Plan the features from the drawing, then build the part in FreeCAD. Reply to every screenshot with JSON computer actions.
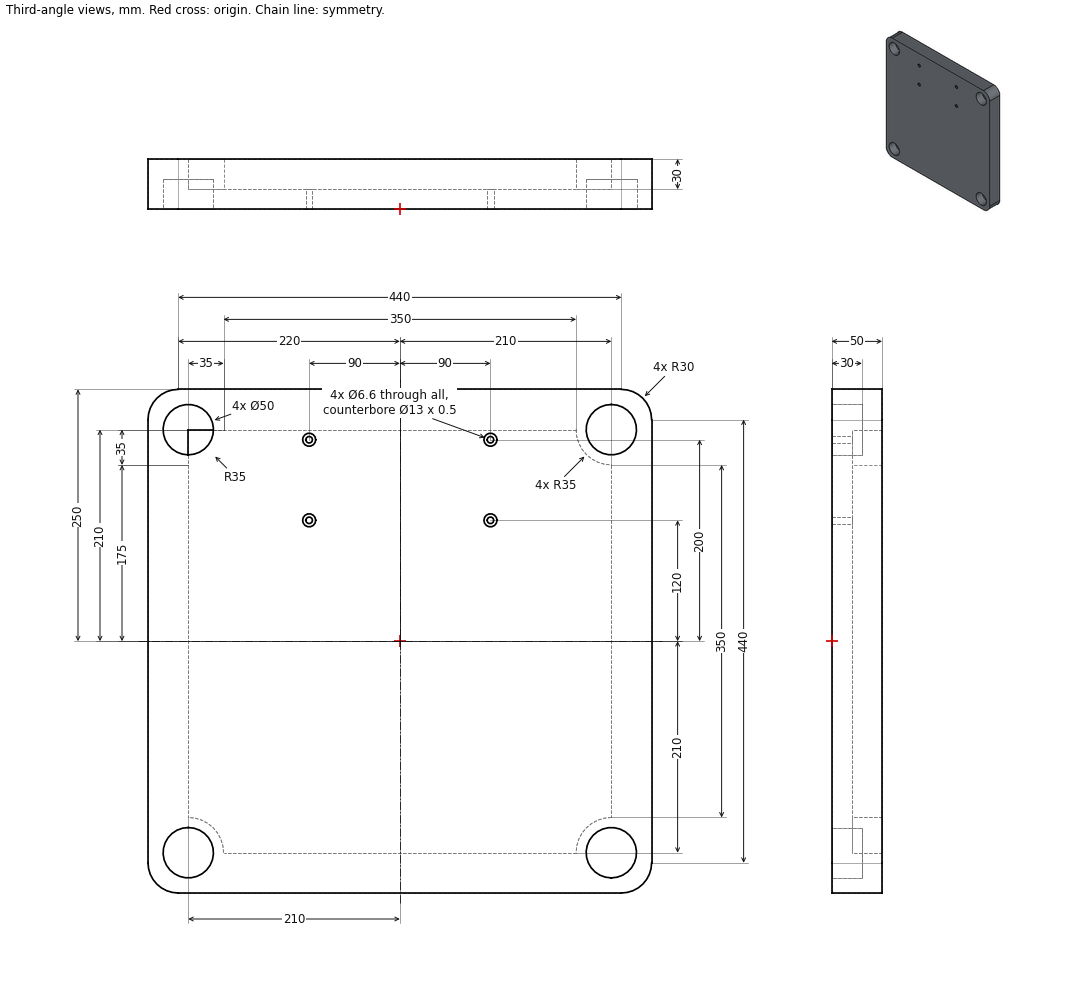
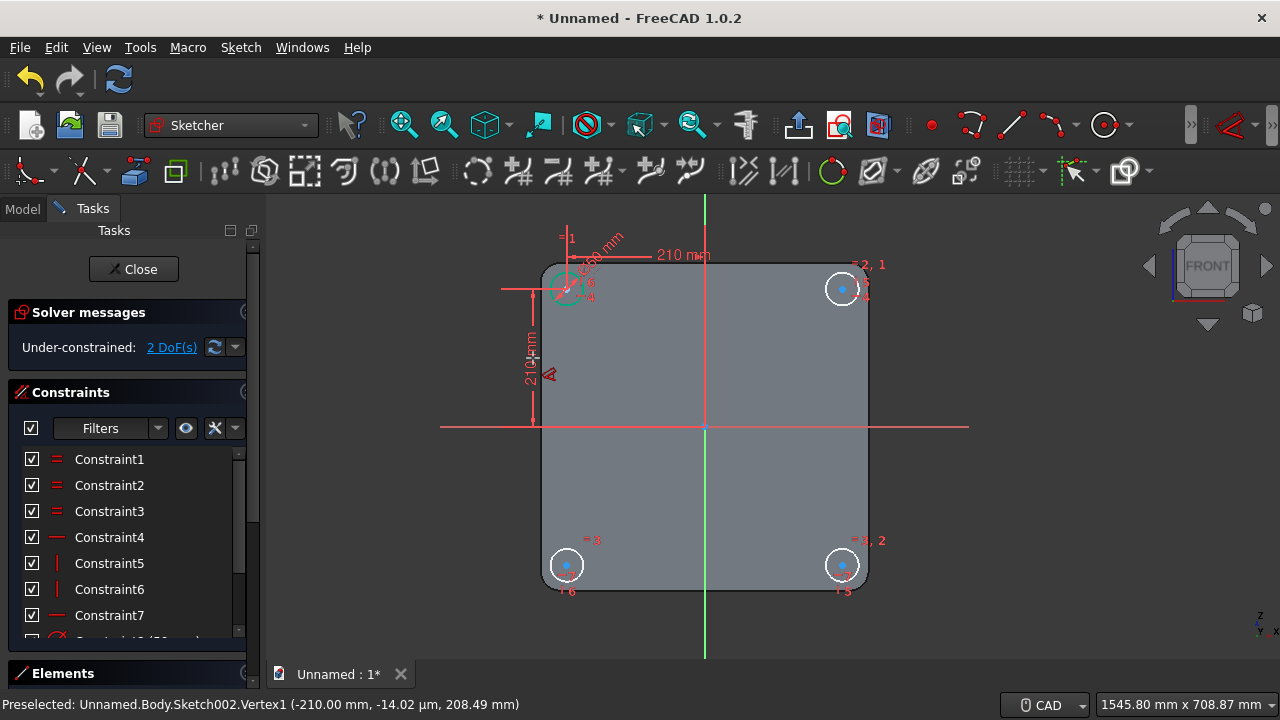
{"action": "left_click", "coordinate": [842, 289]}
{"action": "left_click", "coordinate": [773, 255]}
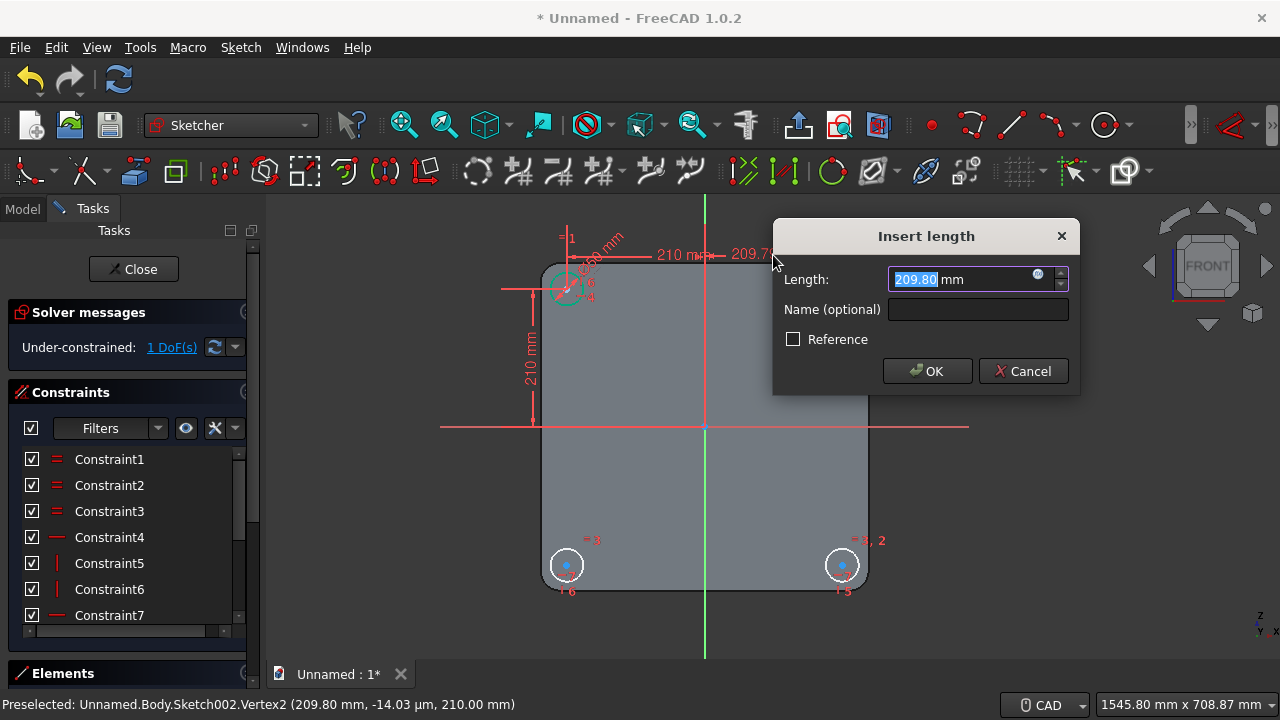
{"action": "type", "text": "210"}
{"action": "key", "text": "Return"}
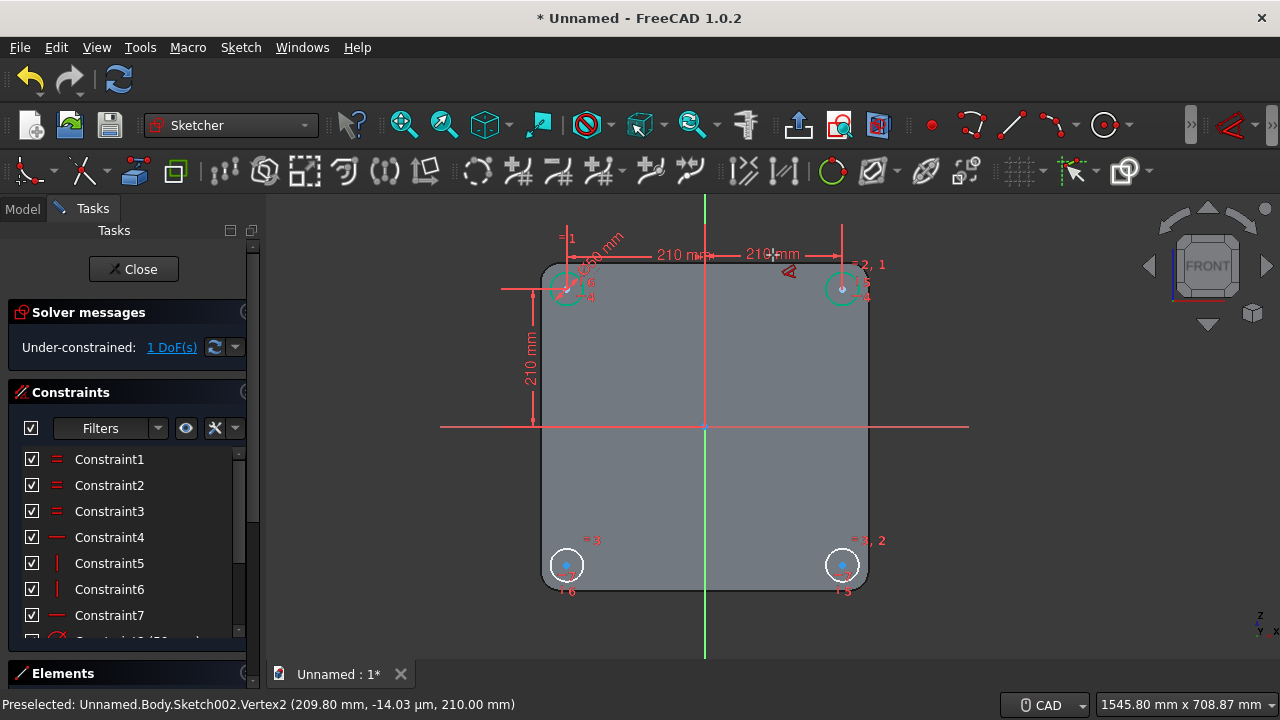
{"action": "left_click", "coordinate": [842, 565]}
{"action": "left_click", "coordinate": [876, 496]}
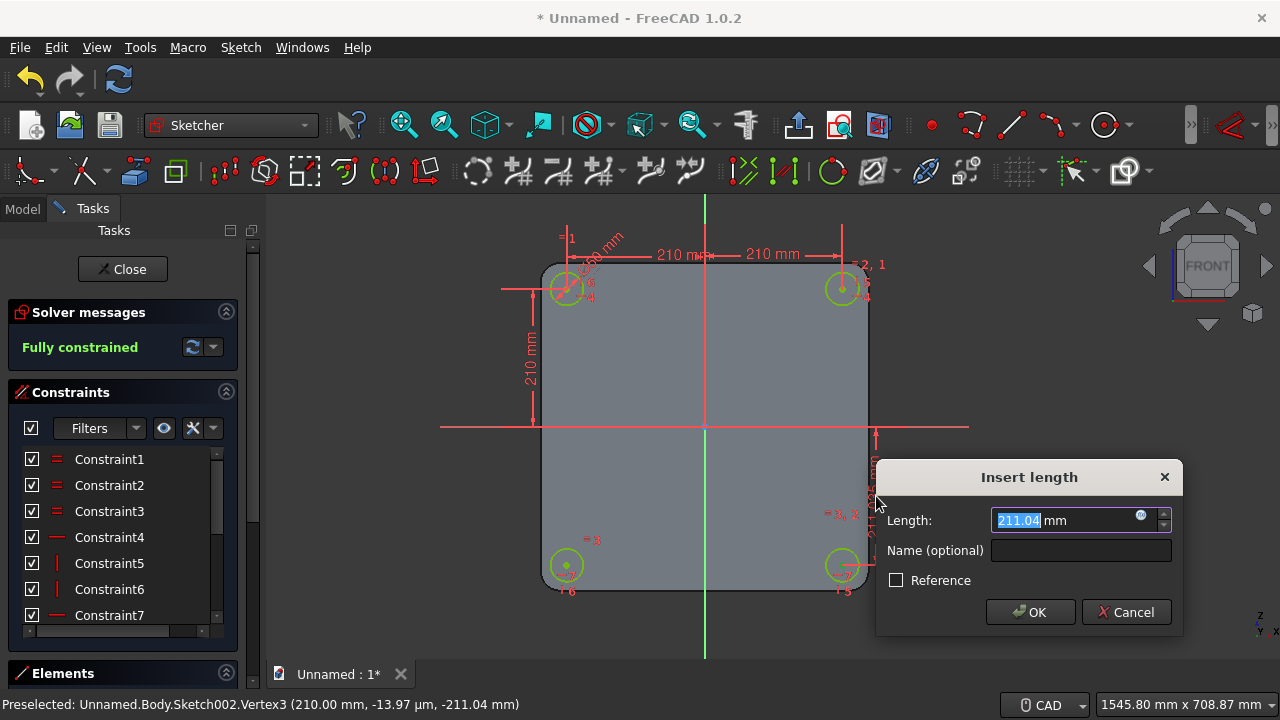
{"action": "type", "text": "210"}
{"action": "key", "text": "Return"}
{"action": "key", "text": "Escape"}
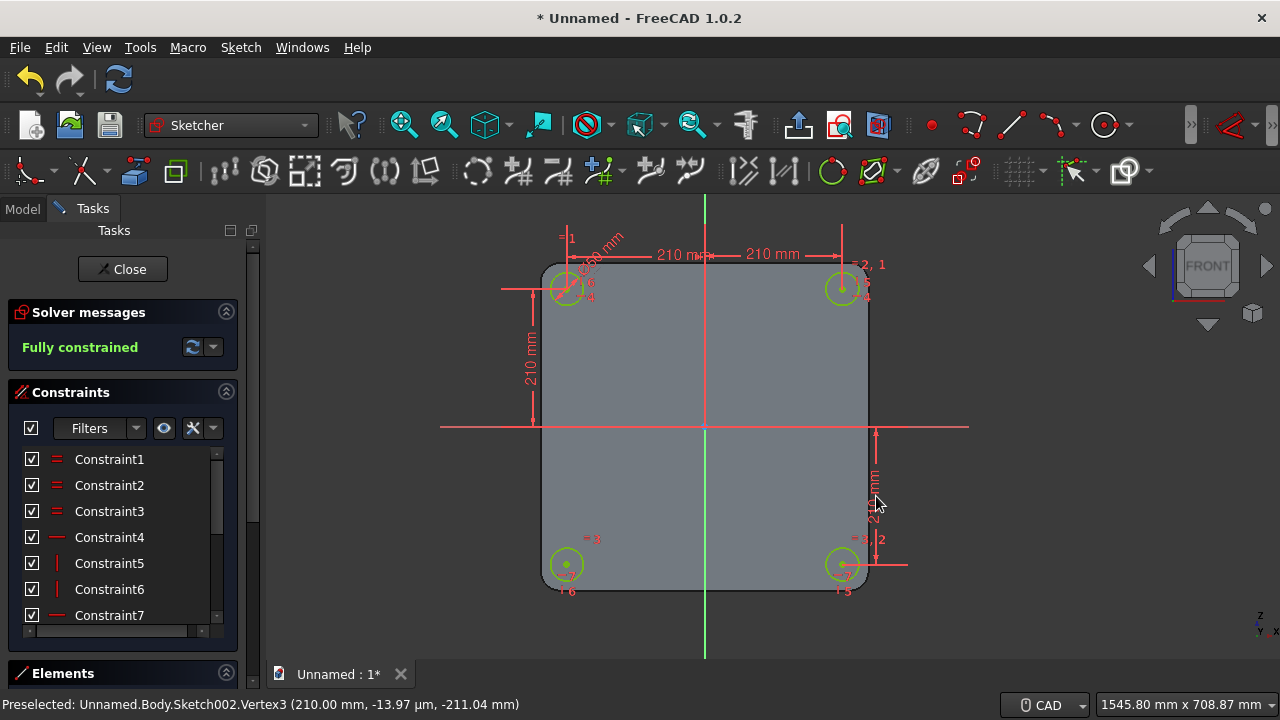
{"action": "left_click", "coordinate": [123, 269]}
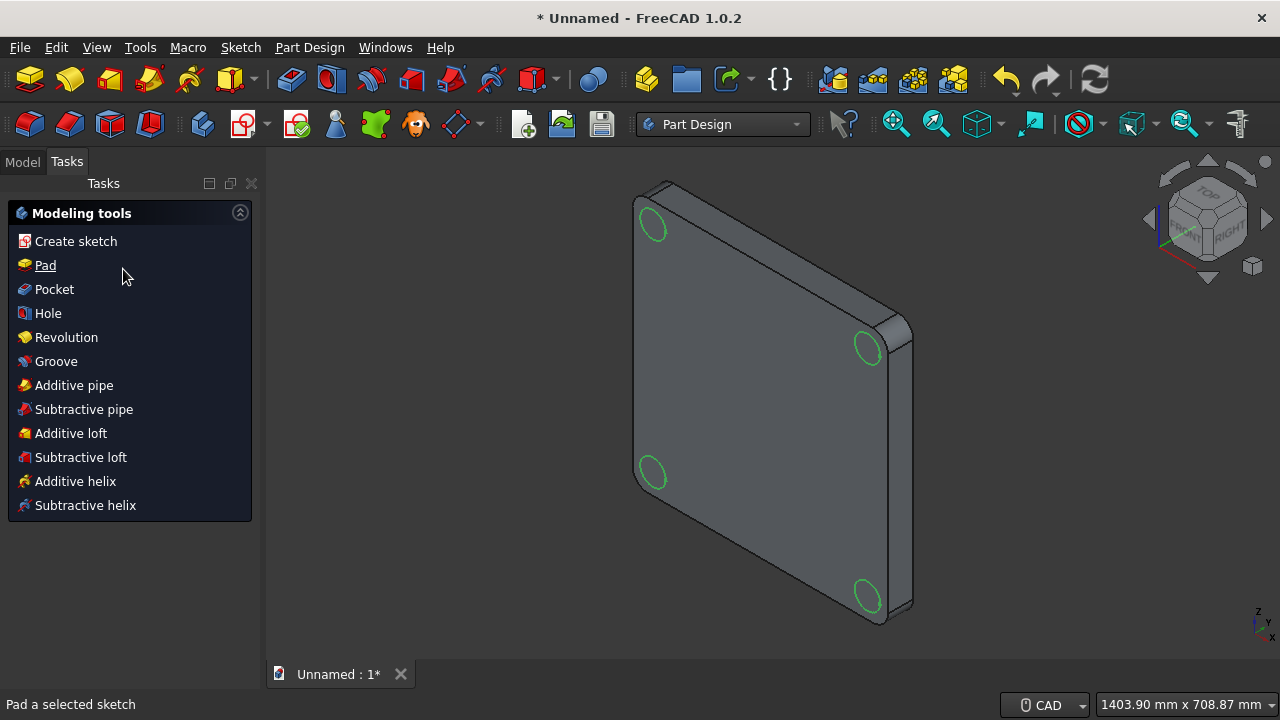
{"action": "left_click", "coordinate": [292, 80]}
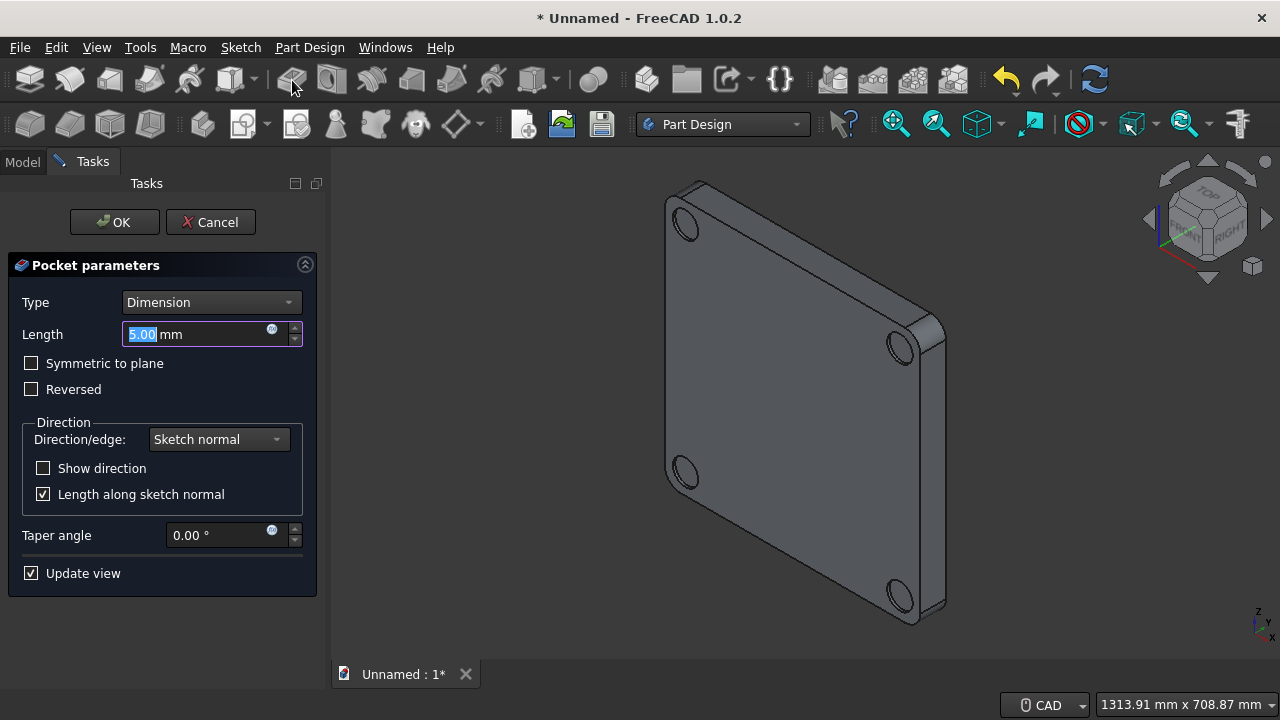
{"action": "type", "text": "30"}
{"action": "key", "text": "Tab"}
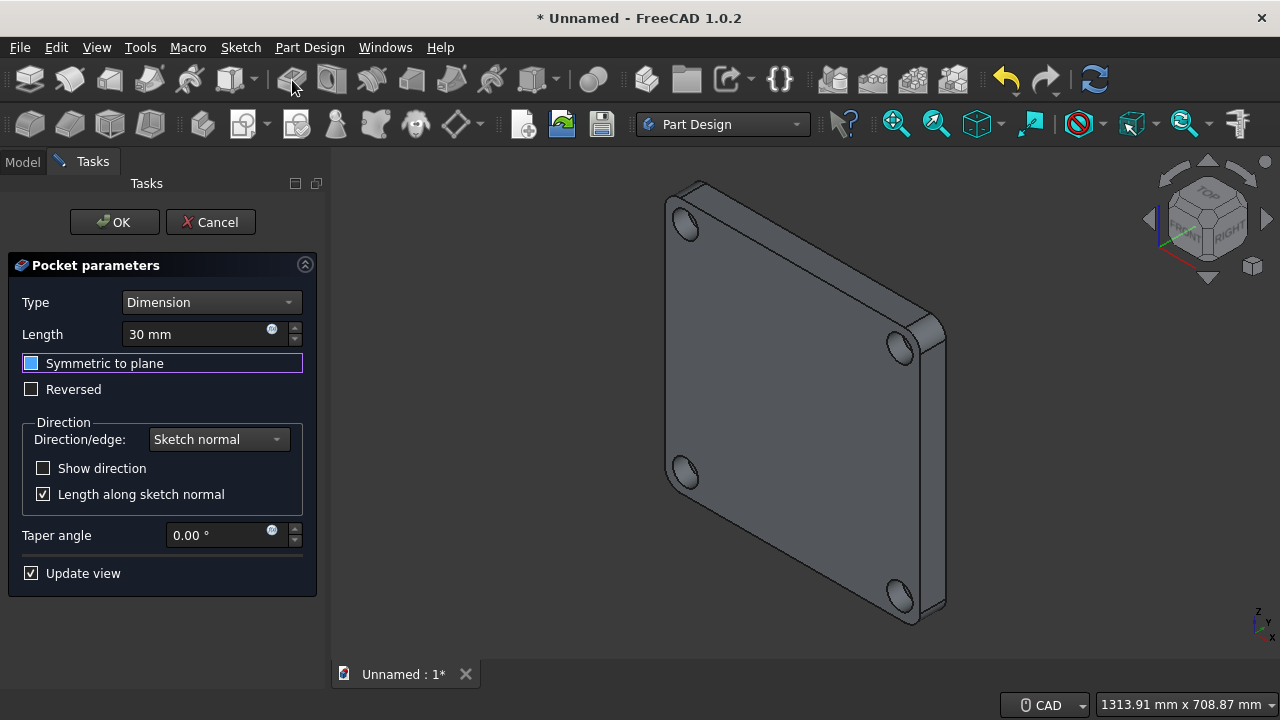
{"action": "left_click", "coordinate": [115, 222]}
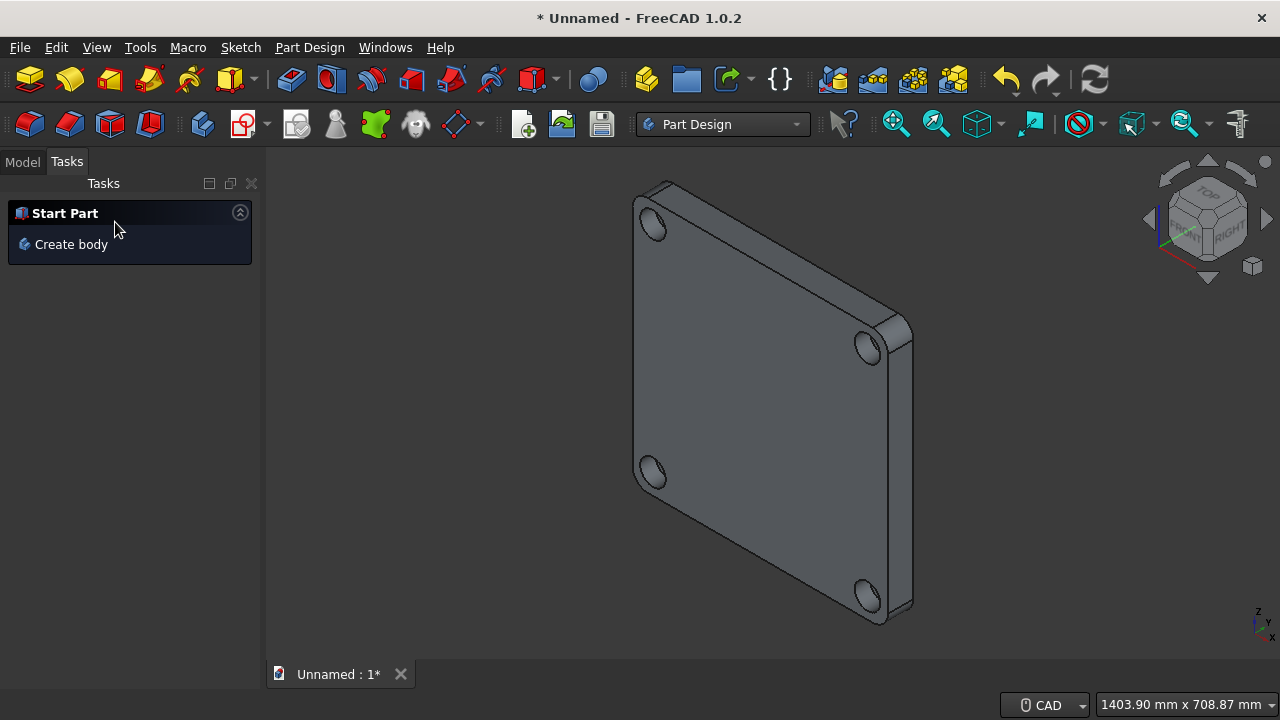
{"action": "left_click", "coordinate": [244, 124]}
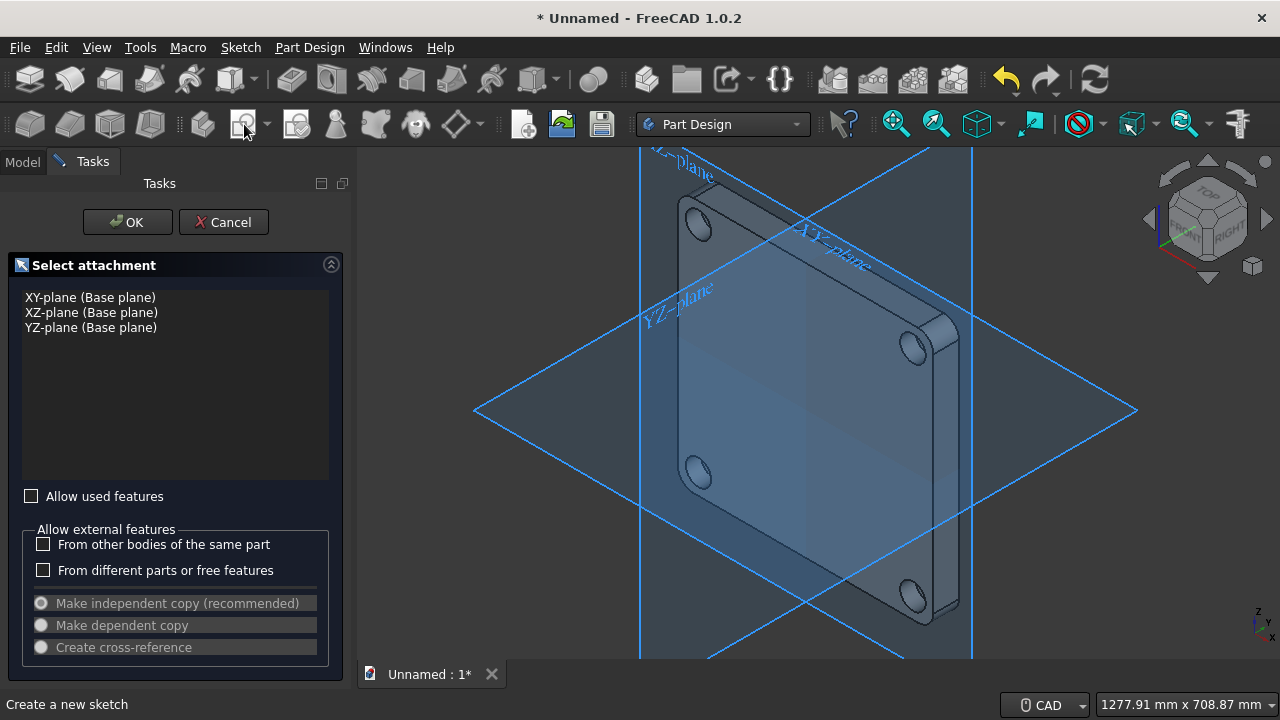
{"action": "left_click", "coordinate": [82, 312]}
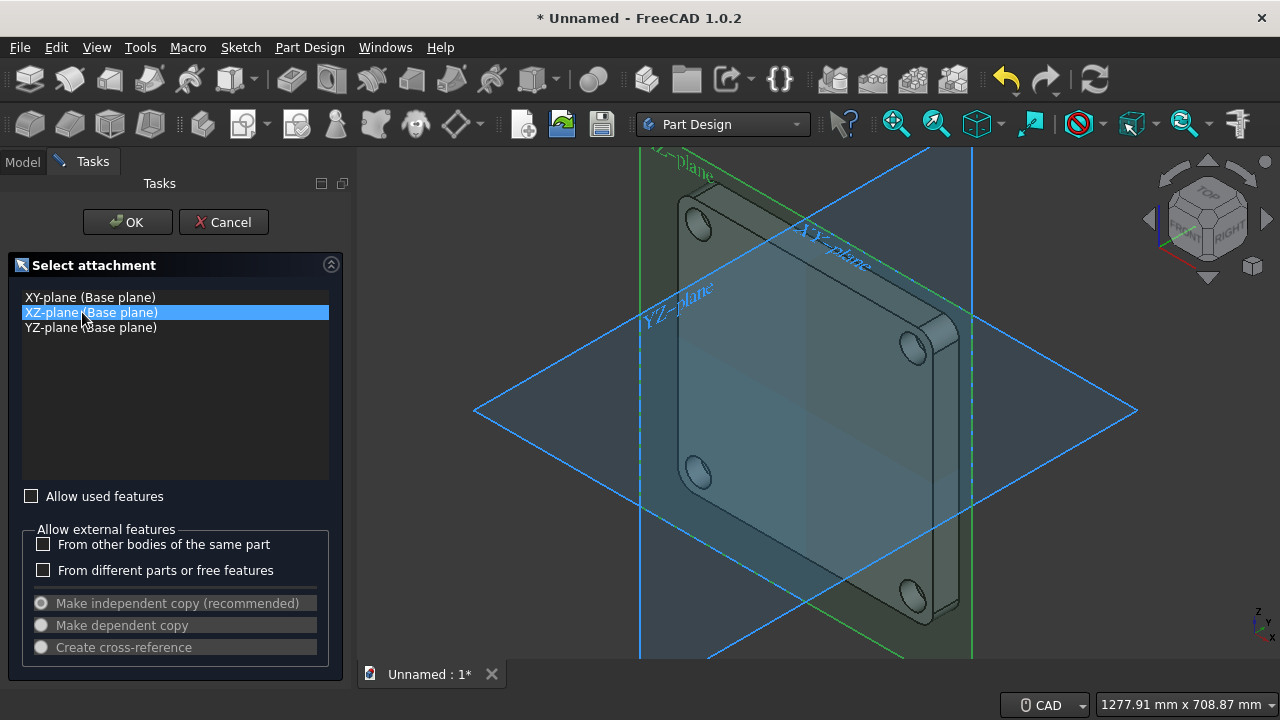
{"action": "left_click", "coordinate": [128, 222]}